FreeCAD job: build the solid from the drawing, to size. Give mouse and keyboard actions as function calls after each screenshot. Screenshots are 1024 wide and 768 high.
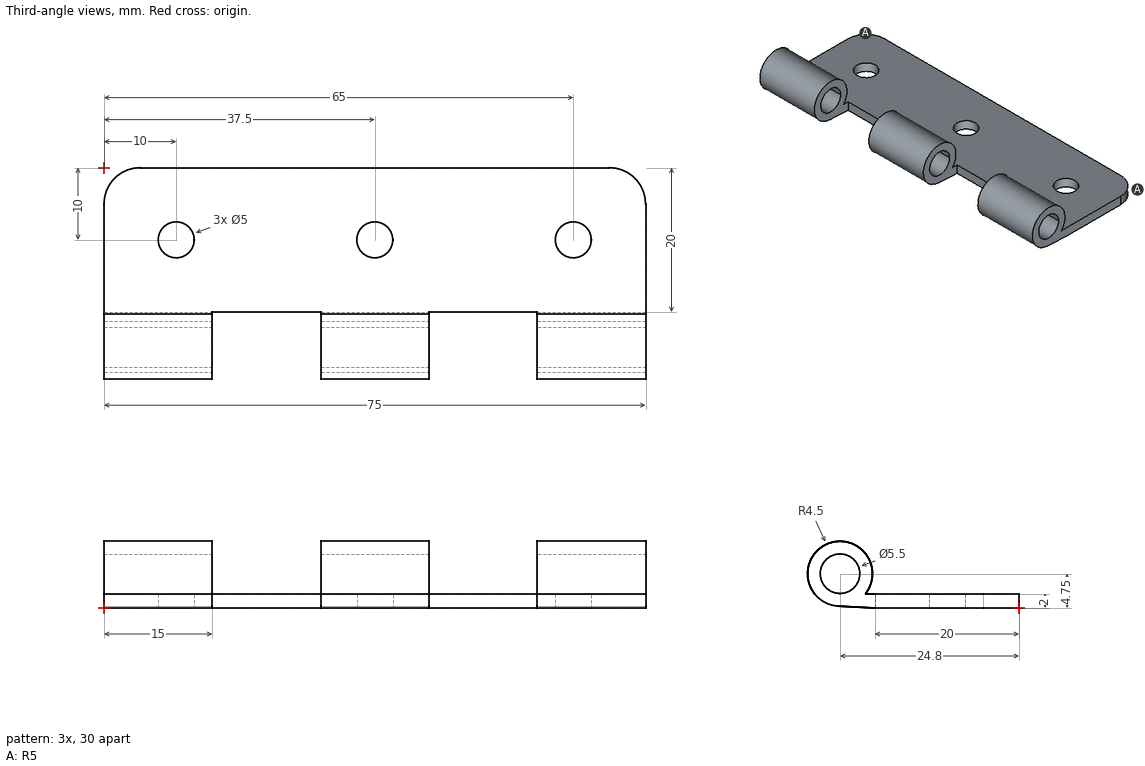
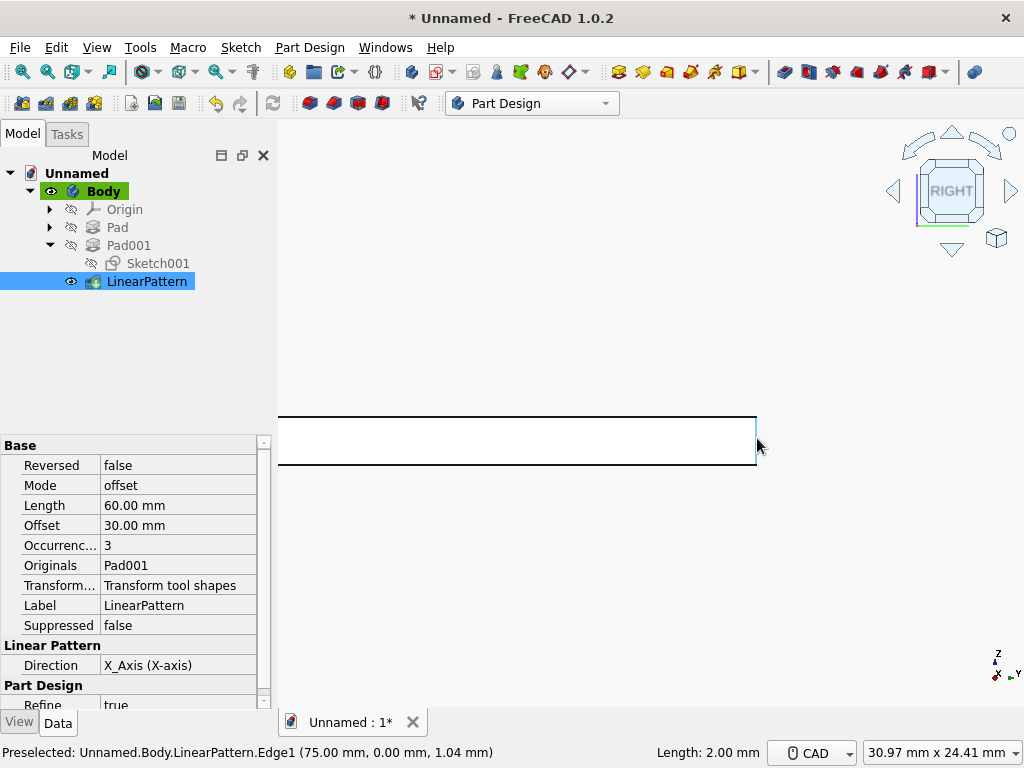
click(24, 72)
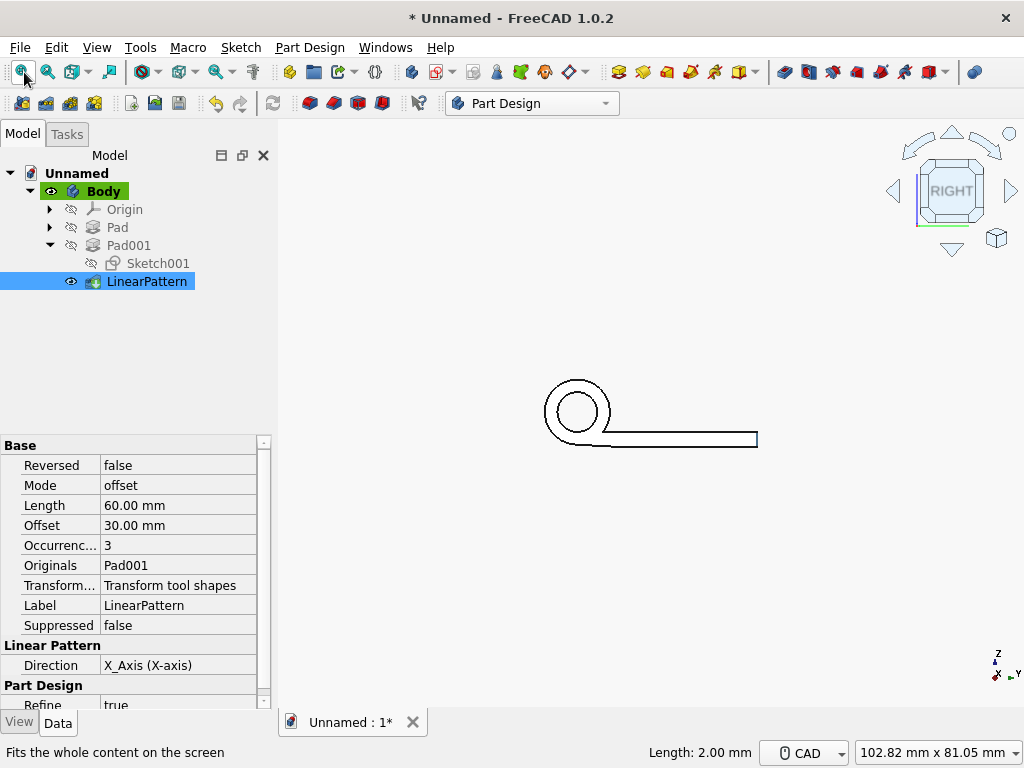
key(5)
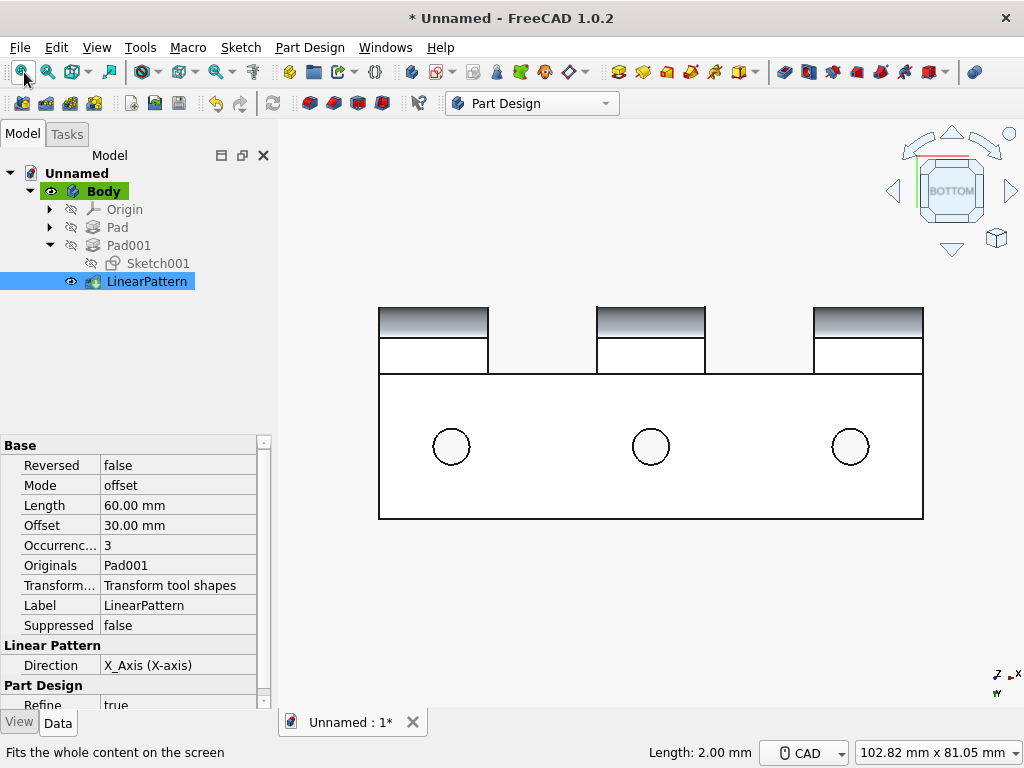
scroll(379, 518, up, 6)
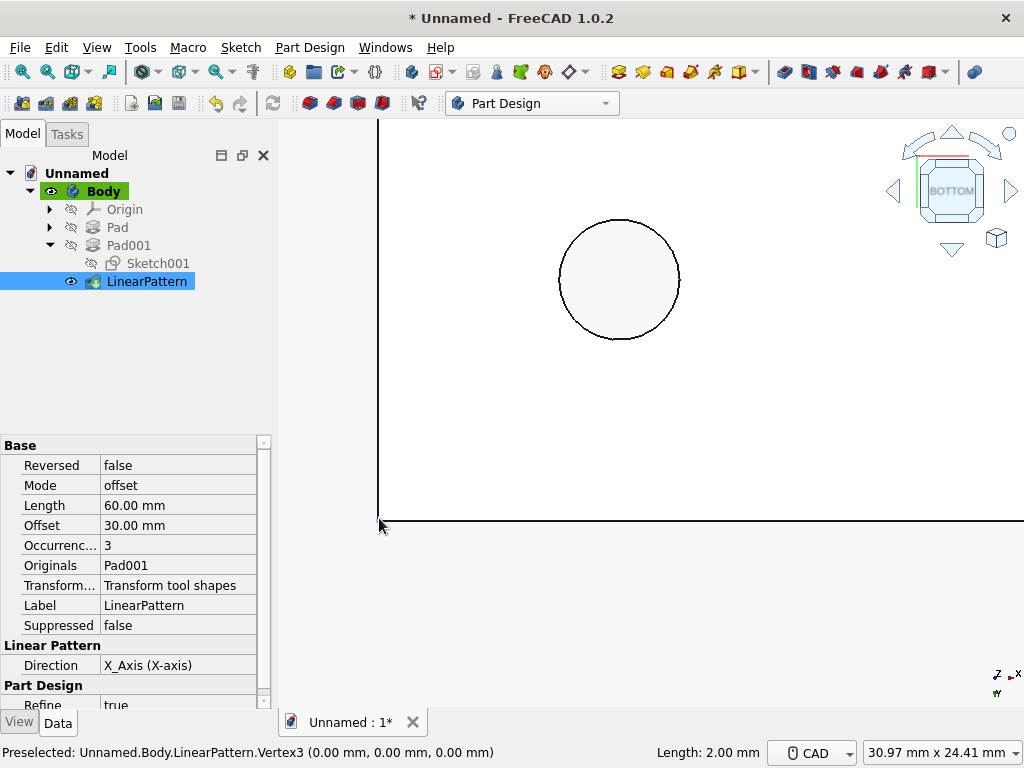
key(v)
key(f)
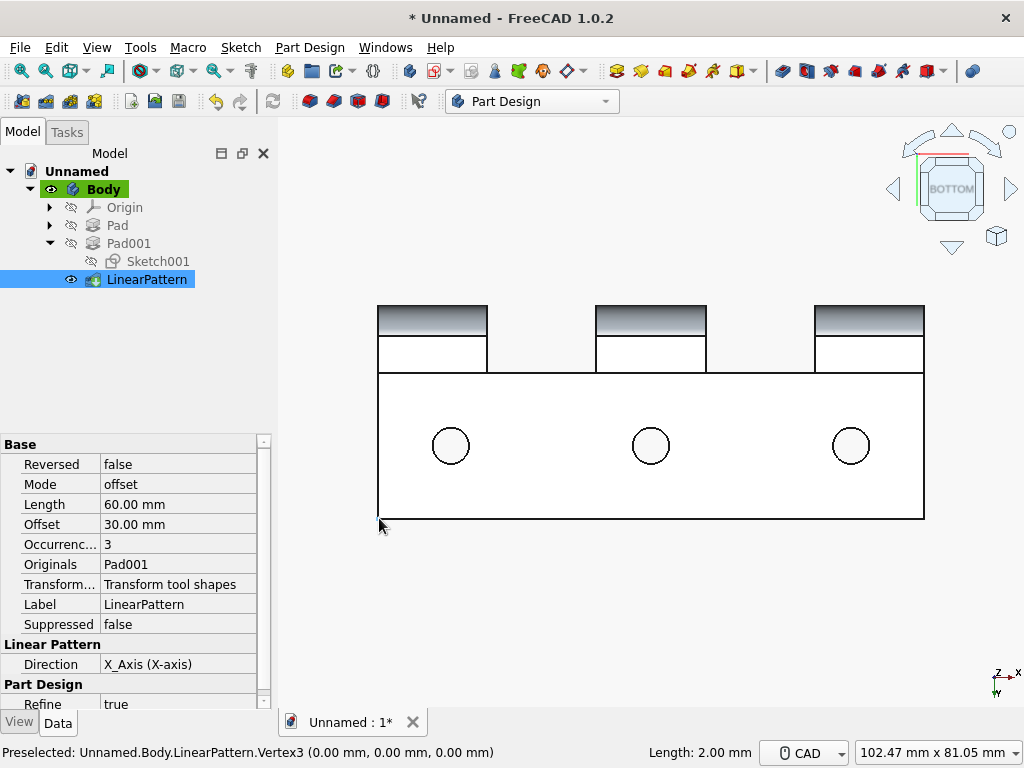
key(4)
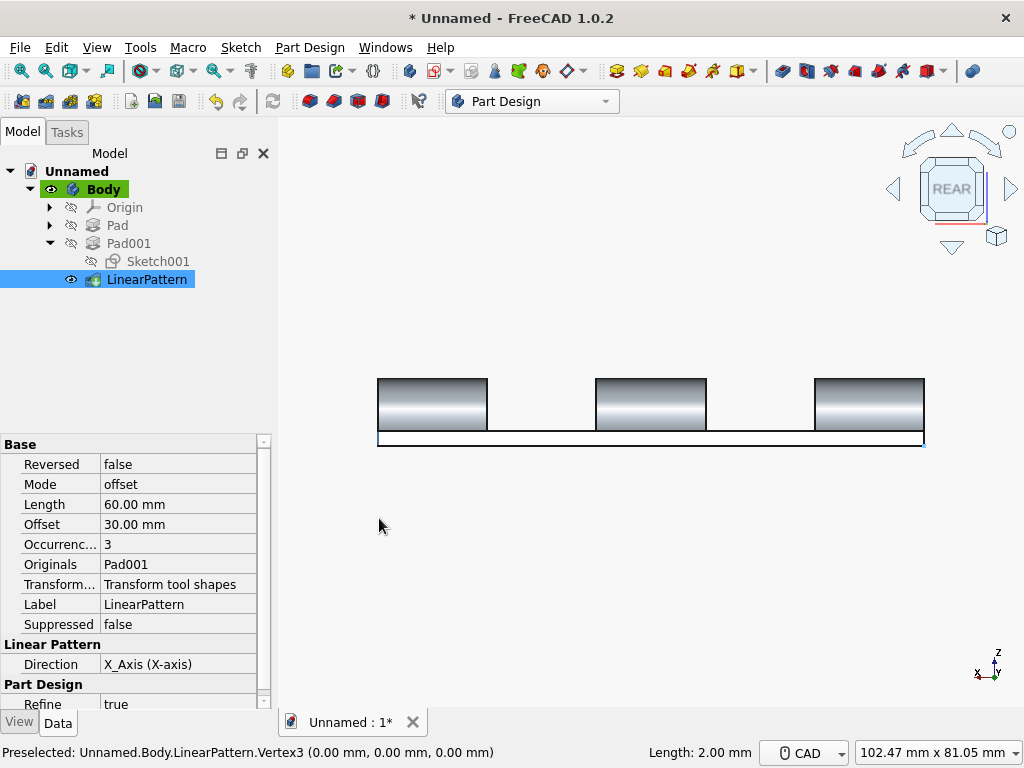
click(924, 437, ctrl)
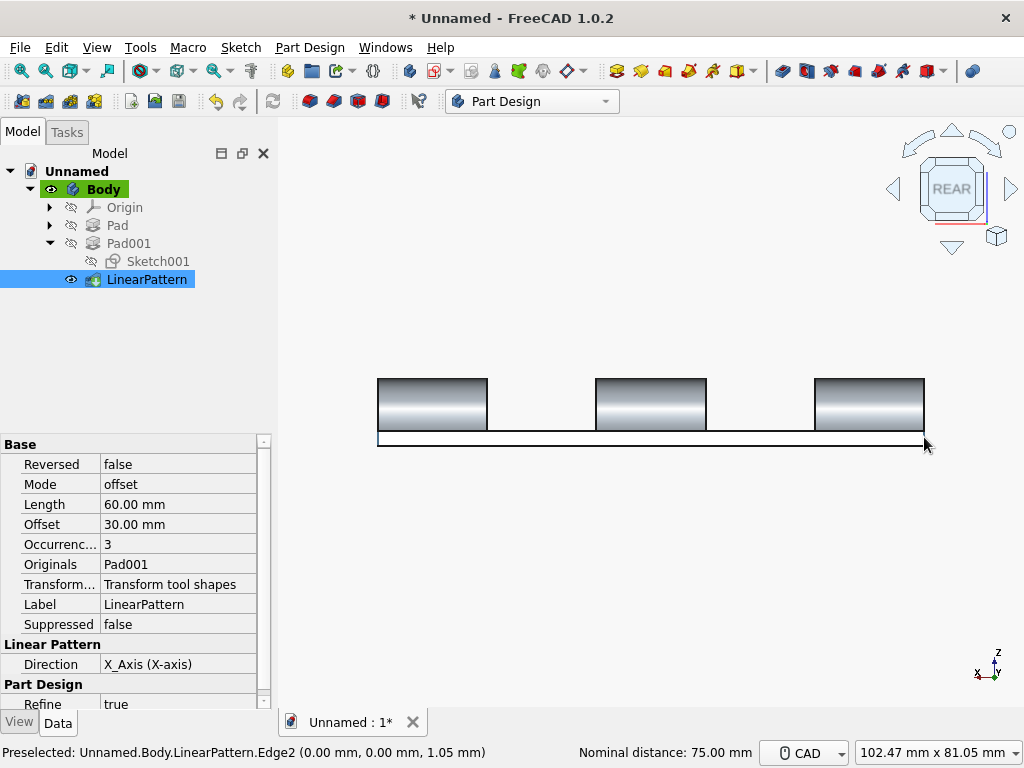
click(310, 102)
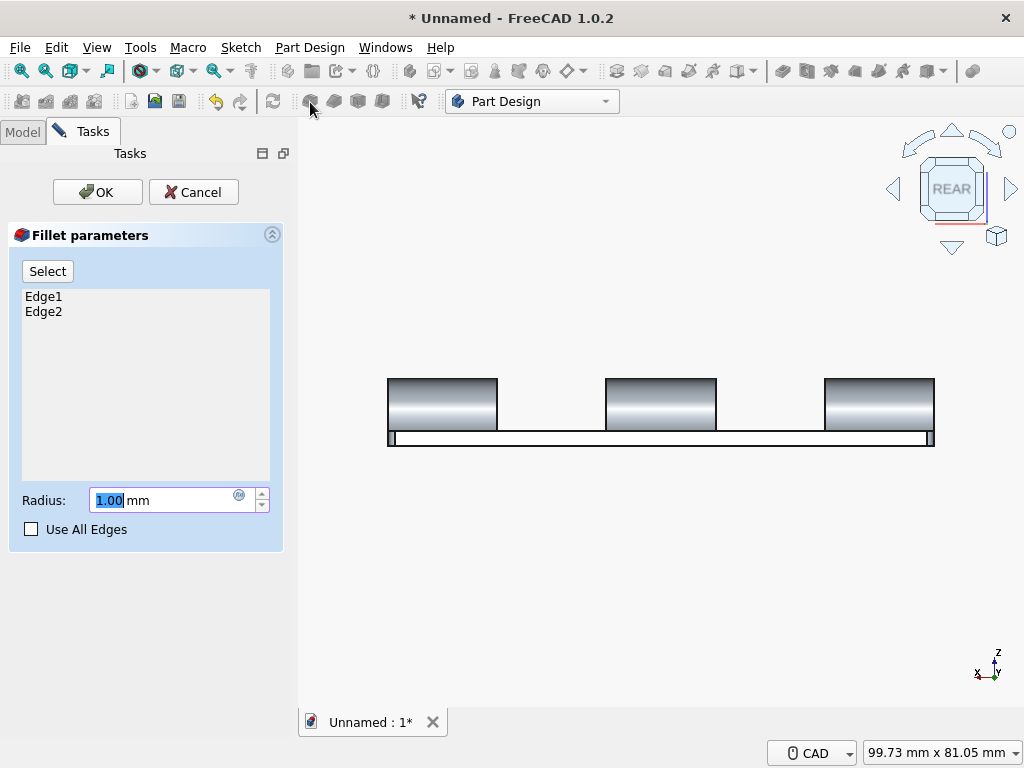
text(5)
key(Tab)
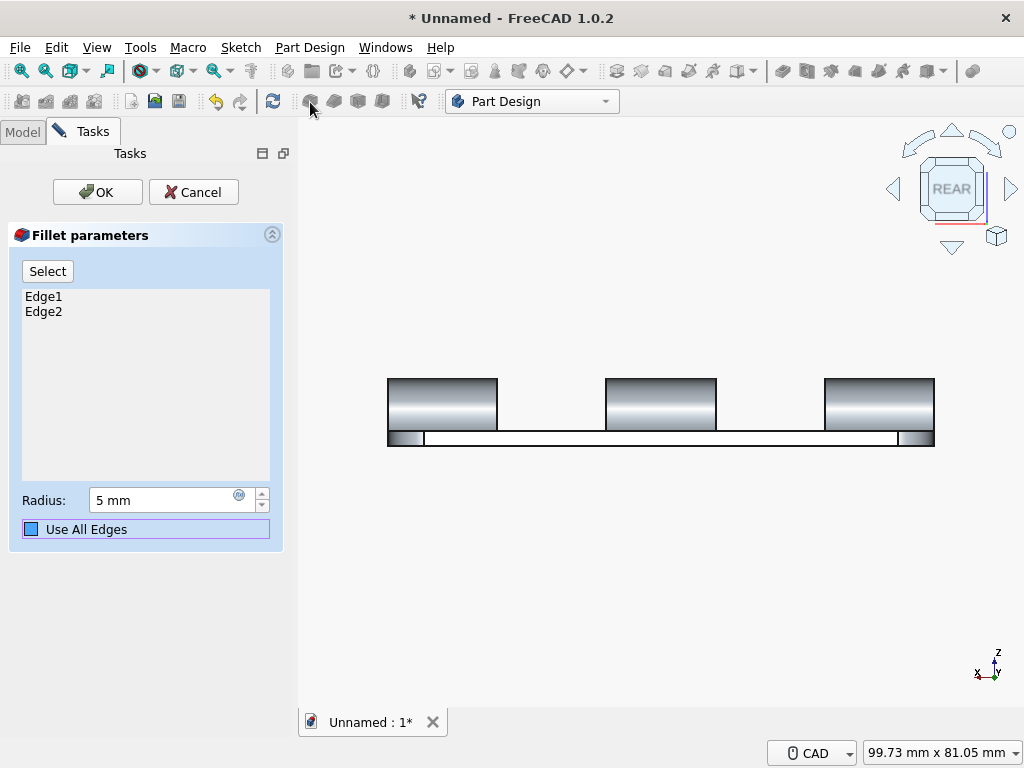
click(98, 192)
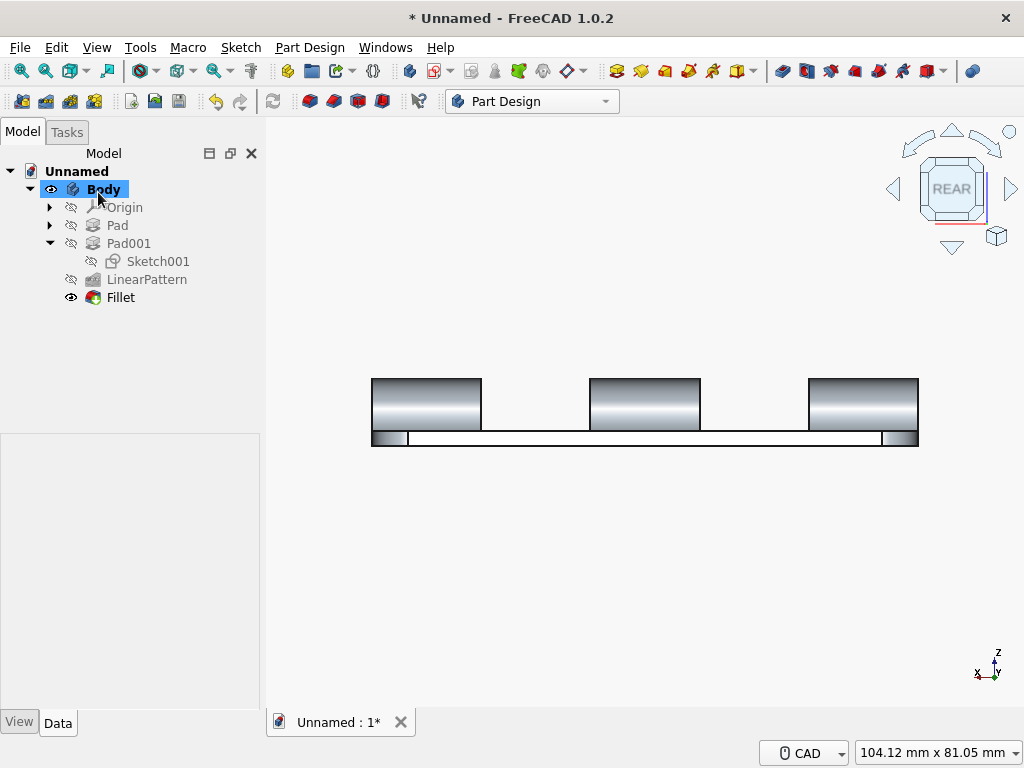
key(0)